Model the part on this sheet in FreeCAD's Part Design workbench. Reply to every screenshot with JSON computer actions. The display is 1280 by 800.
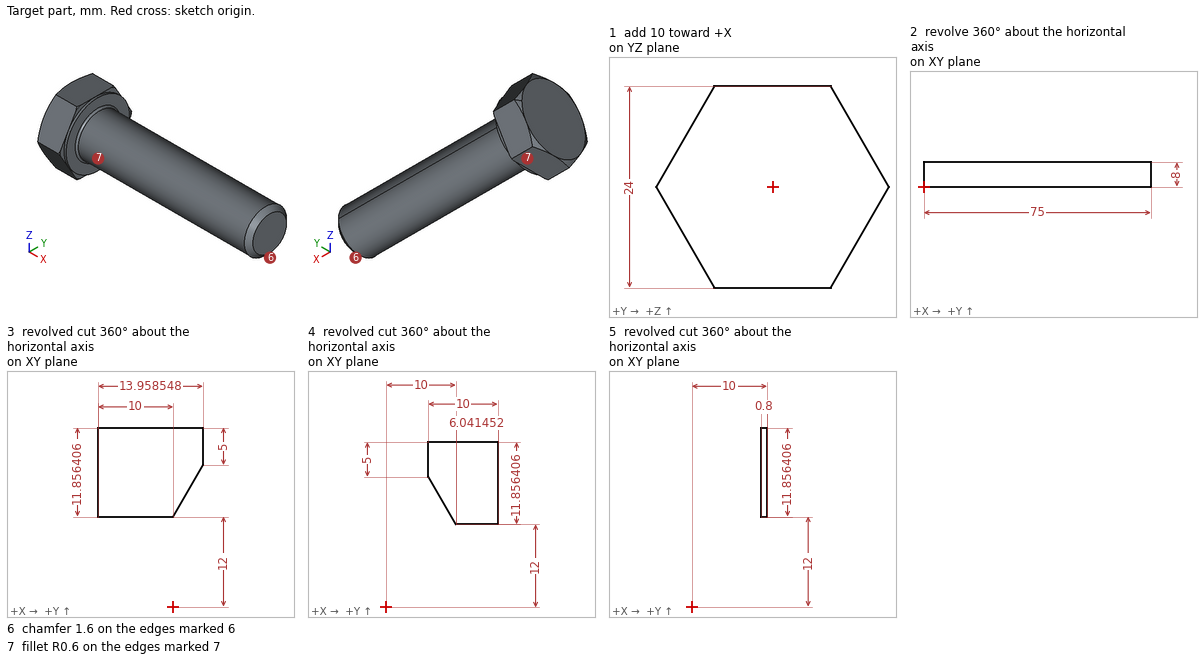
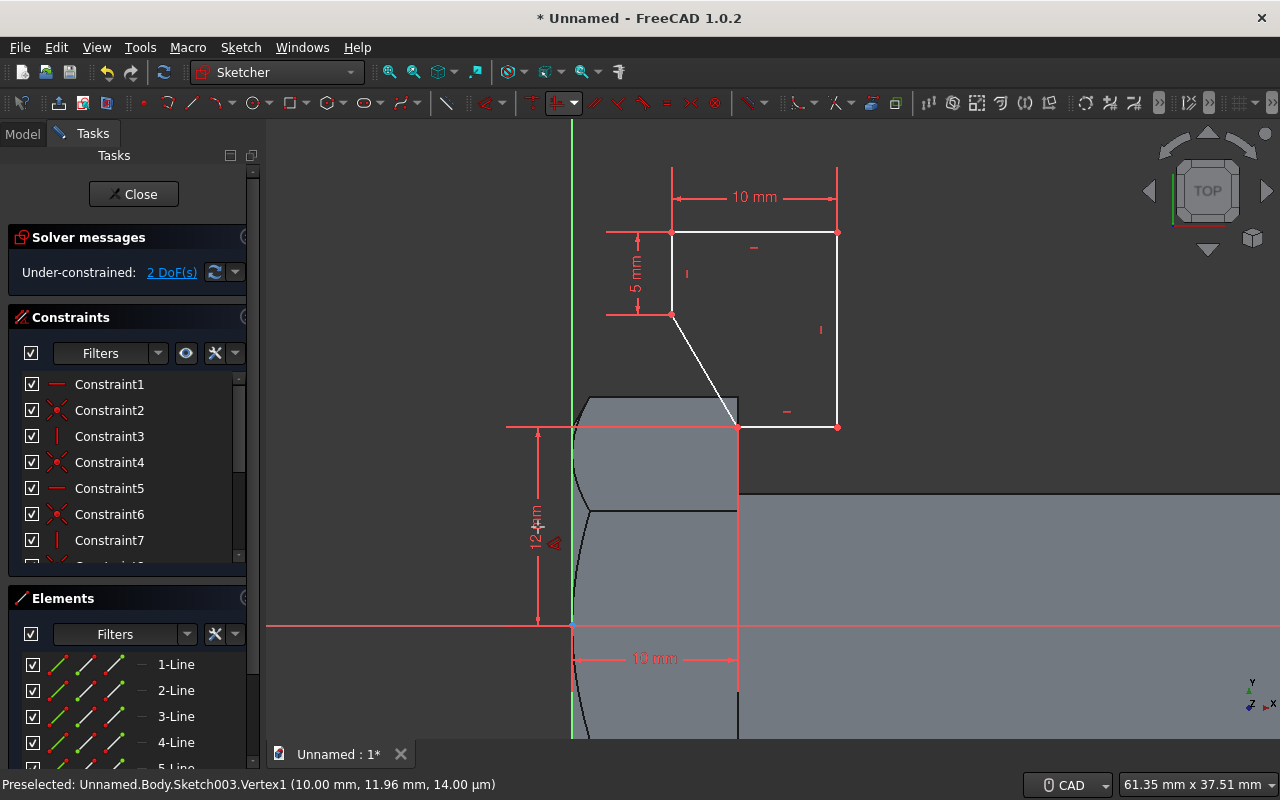
{"action": "left_click", "coordinate": [767, 427]}
{"action": "left_click", "coordinate": [787, 393]}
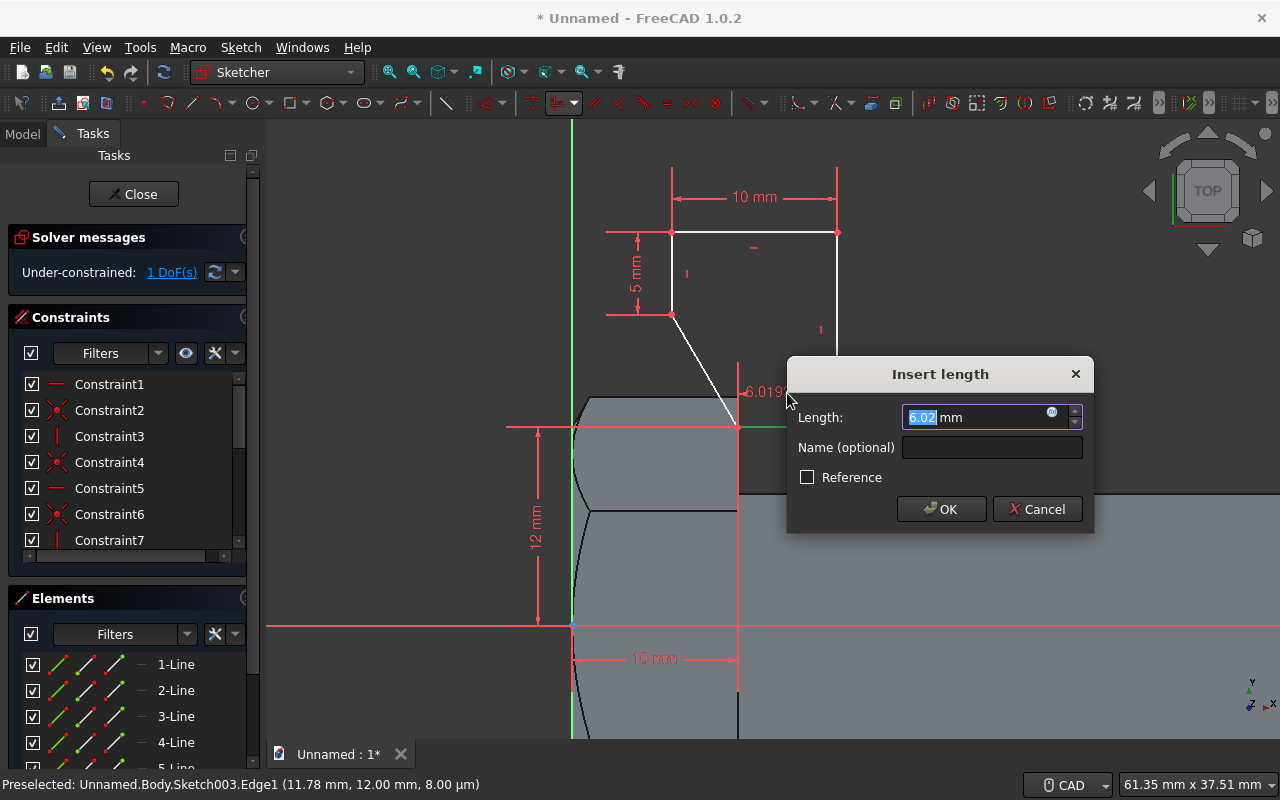
{"action": "type", "text": "6.041452"}
{"action": "key", "text": "Return"}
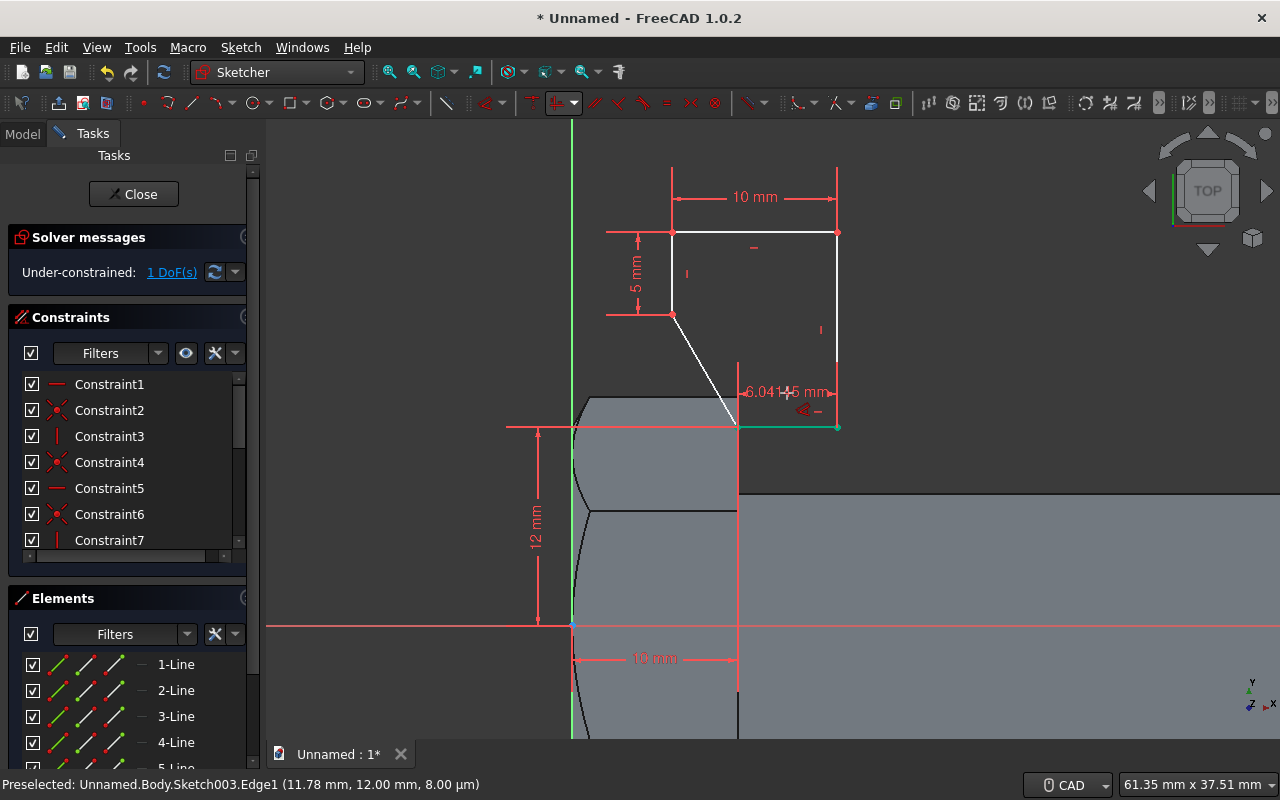
{"action": "left_click", "coordinate": [837, 369]}
{"action": "left_click", "coordinate": [871, 330]}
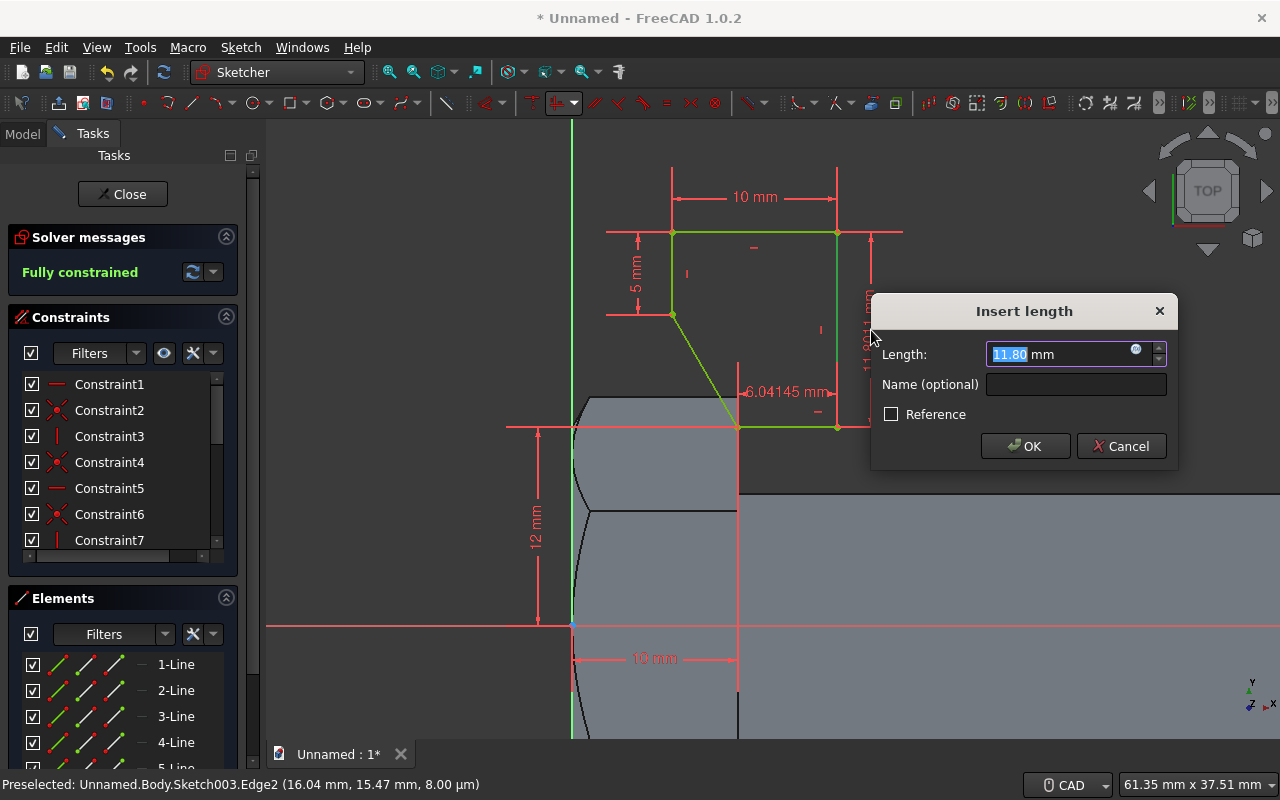
{"action": "type", "text": "11.856406"}
{"action": "key", "text": "Return"}
{"action": "key", "text": "Escape"}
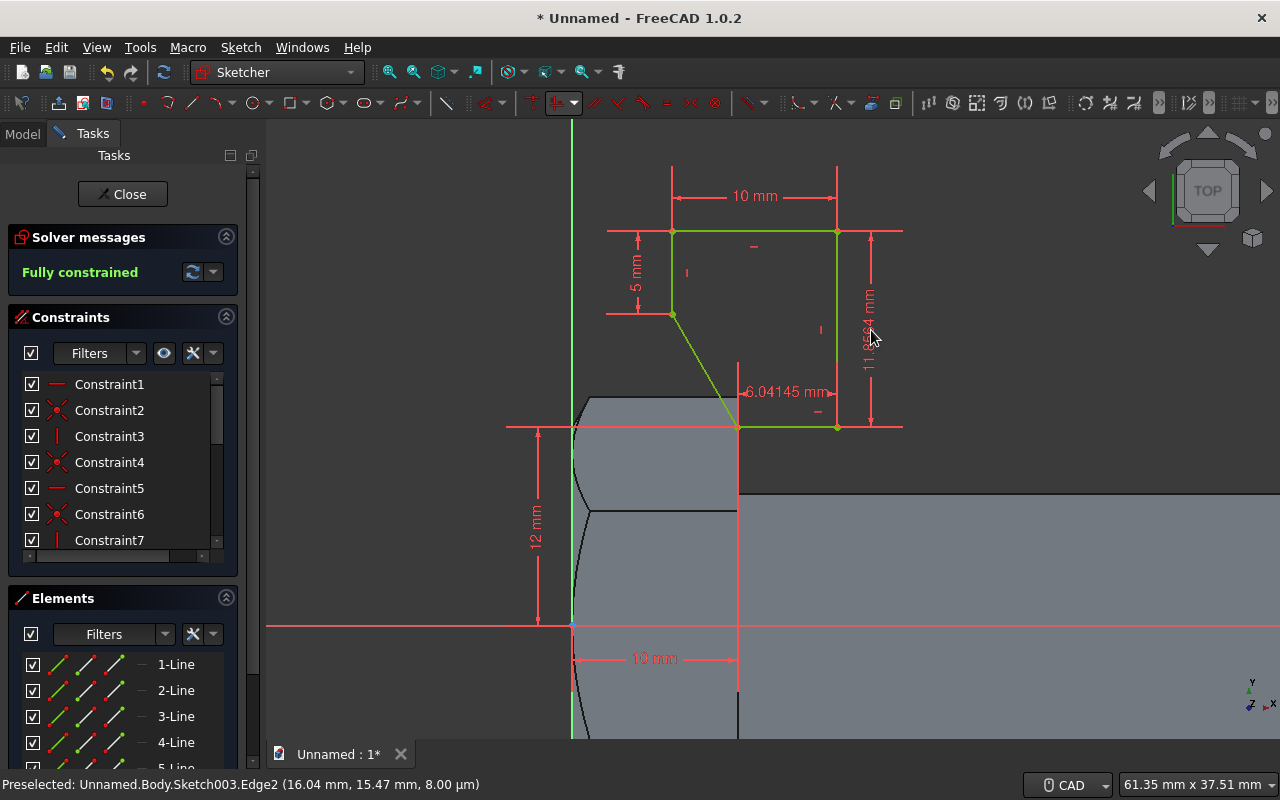
{"action": "left_click", "coordinate": [123, 194]}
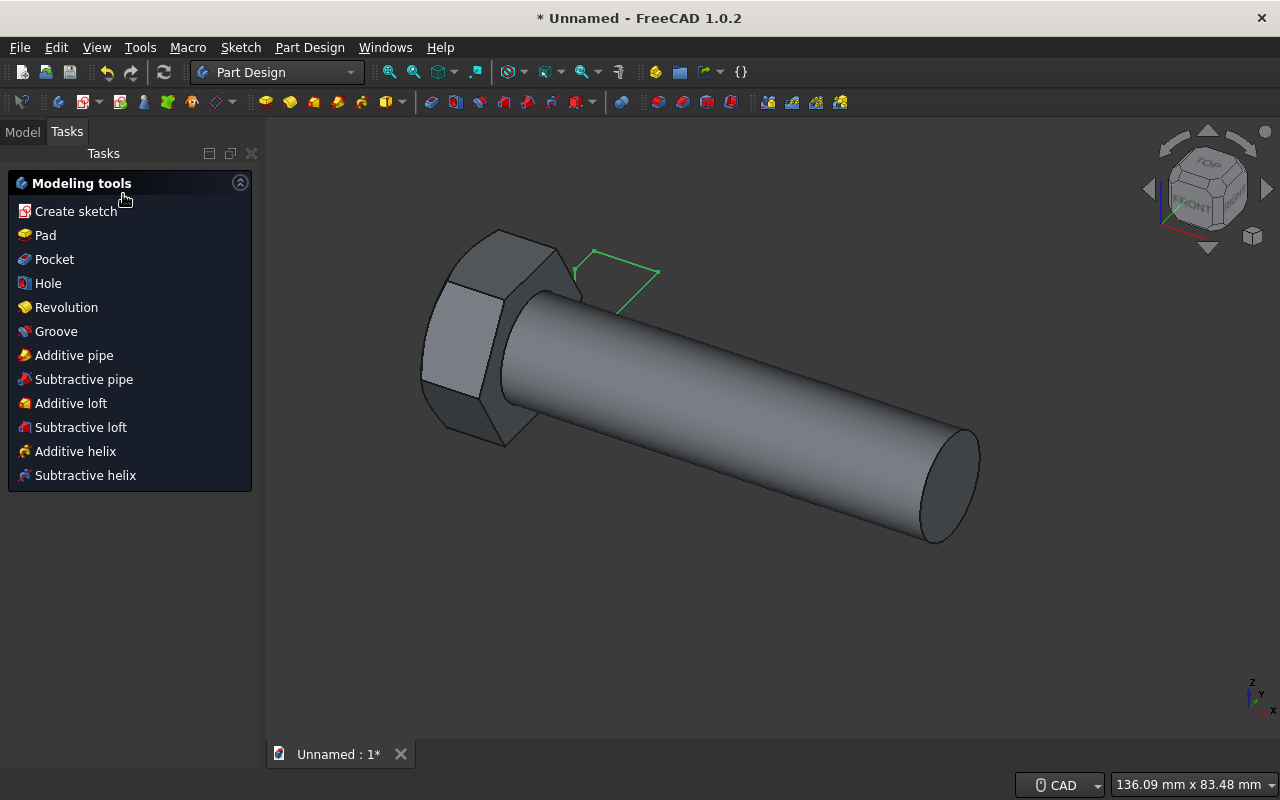
{"action": "left_click", "coordinate": [480, 102]}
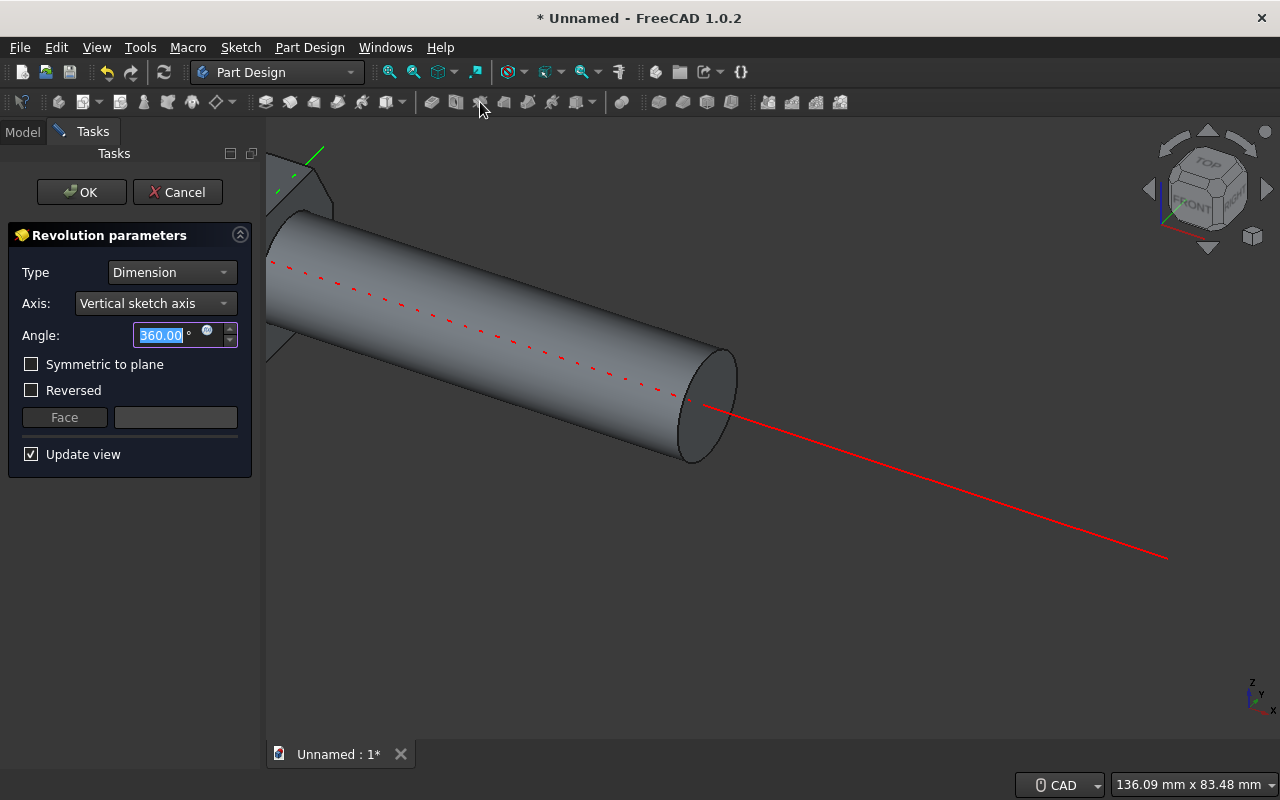
{"action": "left_click", "coordinate": [156, 304]}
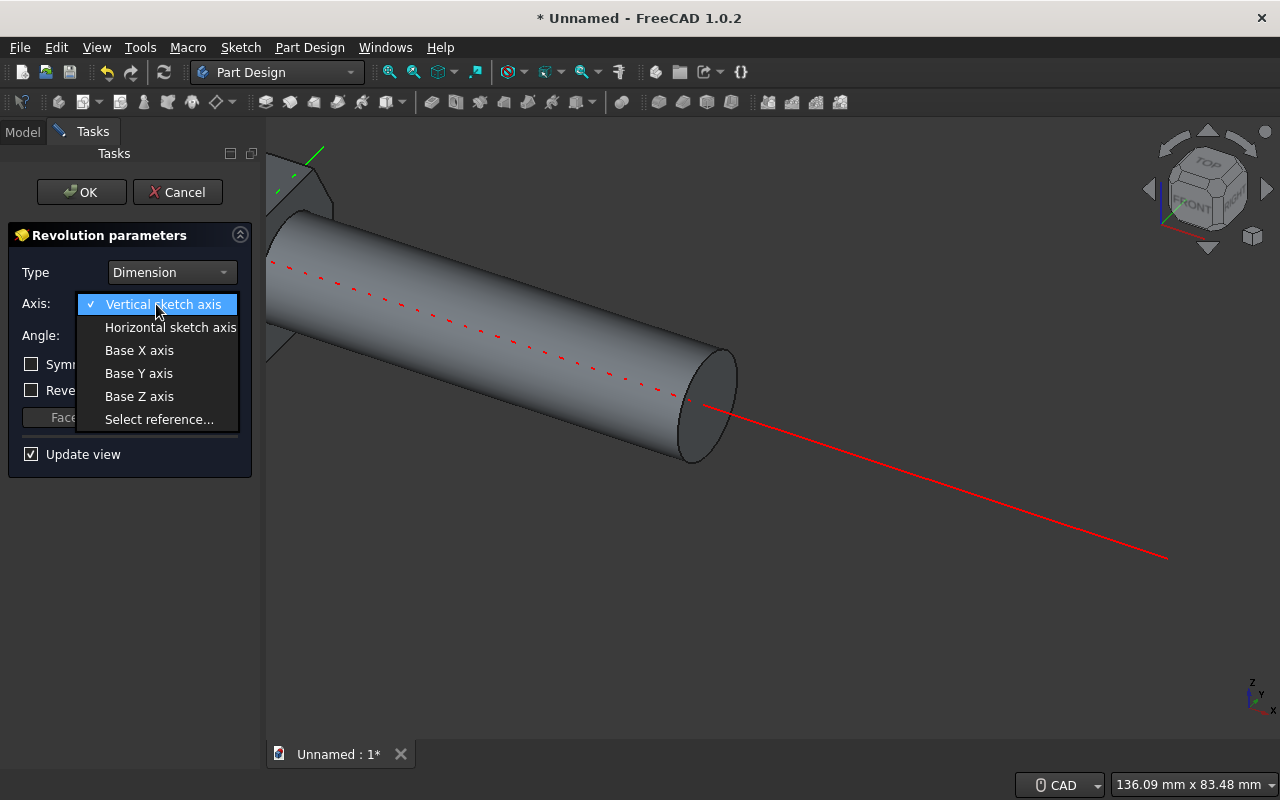
{"action": "left_click", "coordinate": [156, 328]}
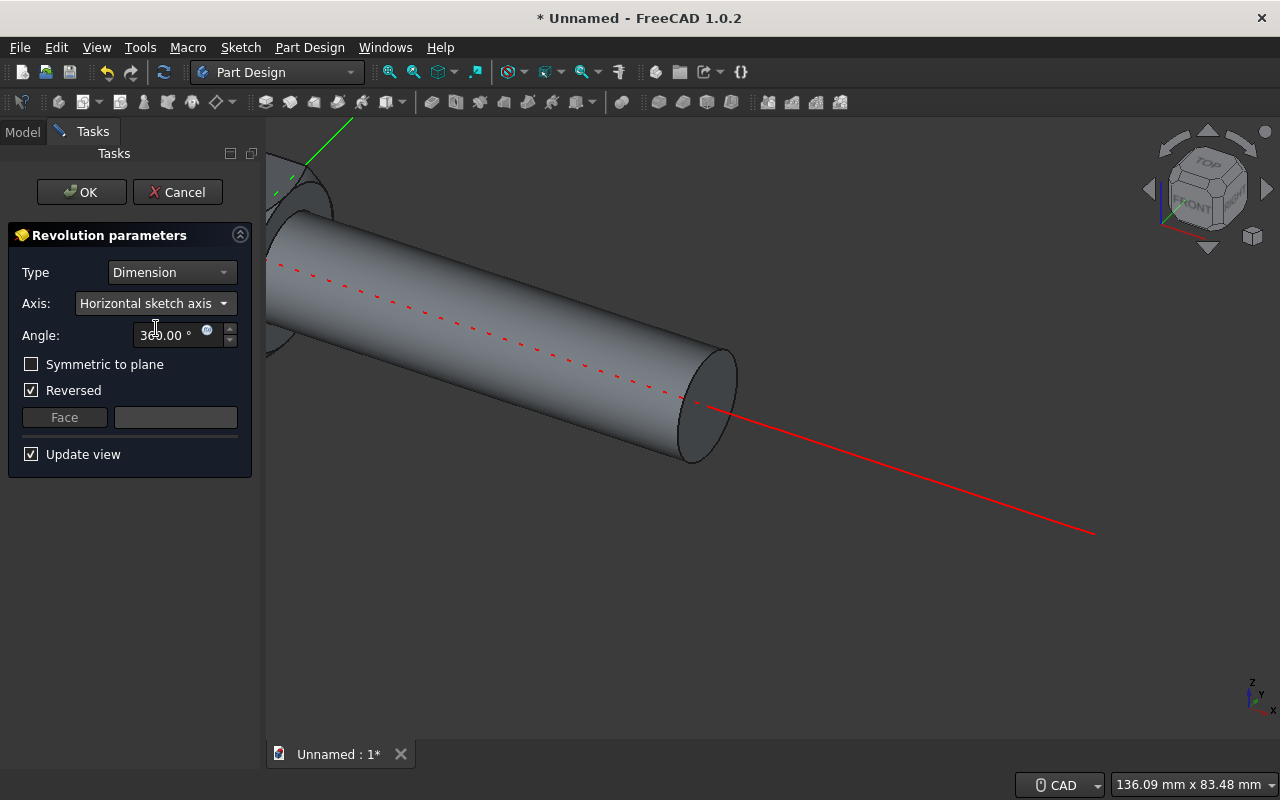
{"action": "left_click", "coordinate": [82, 192]}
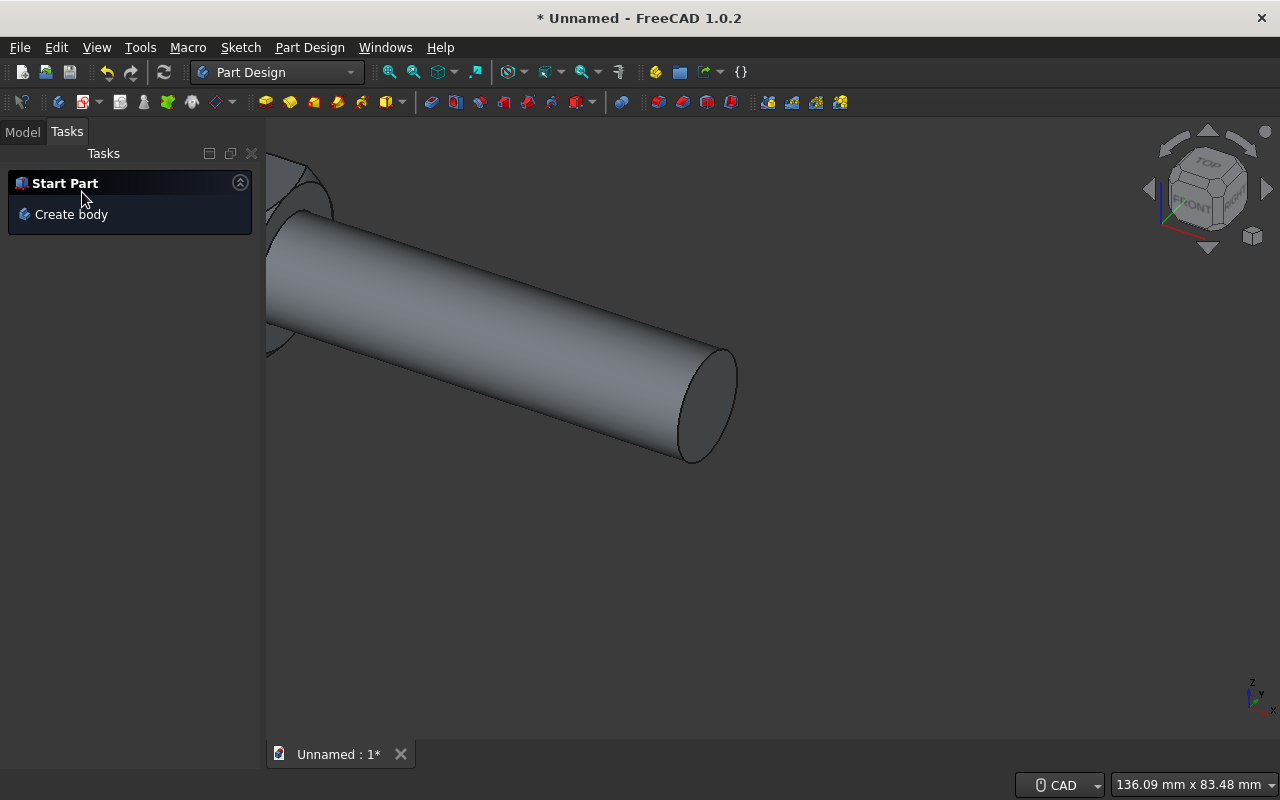
{"action": "left_click", "coordinate": [390, 72]}